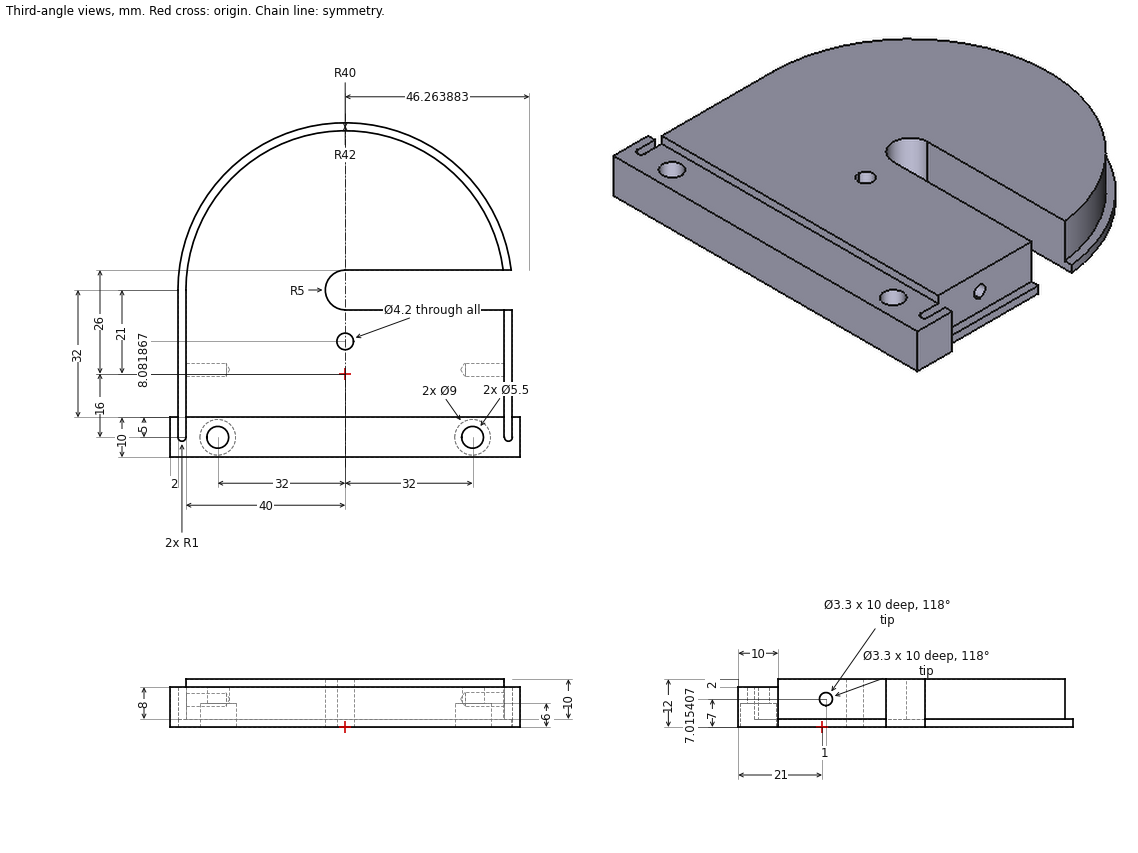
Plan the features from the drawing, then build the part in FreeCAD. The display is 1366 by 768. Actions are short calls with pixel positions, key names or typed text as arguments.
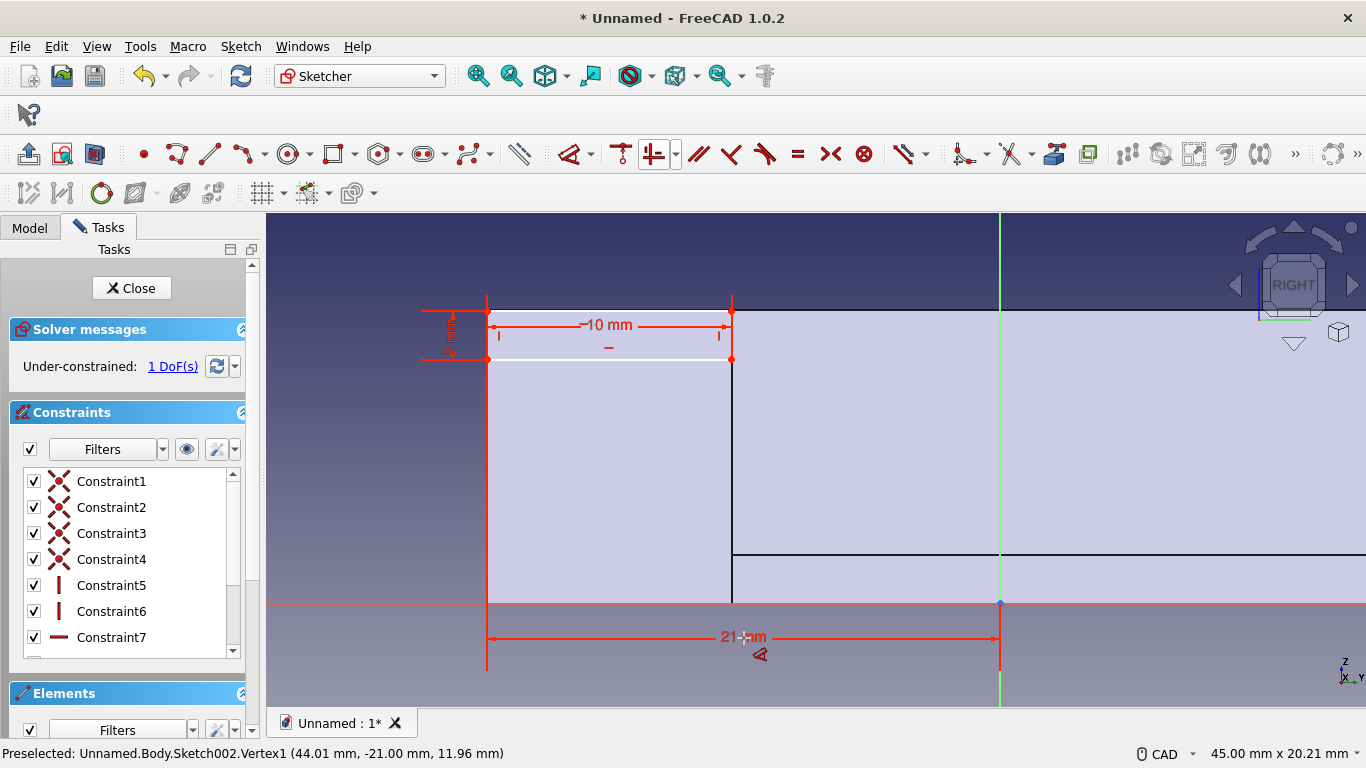
click(487, 311)
click(1034, 457)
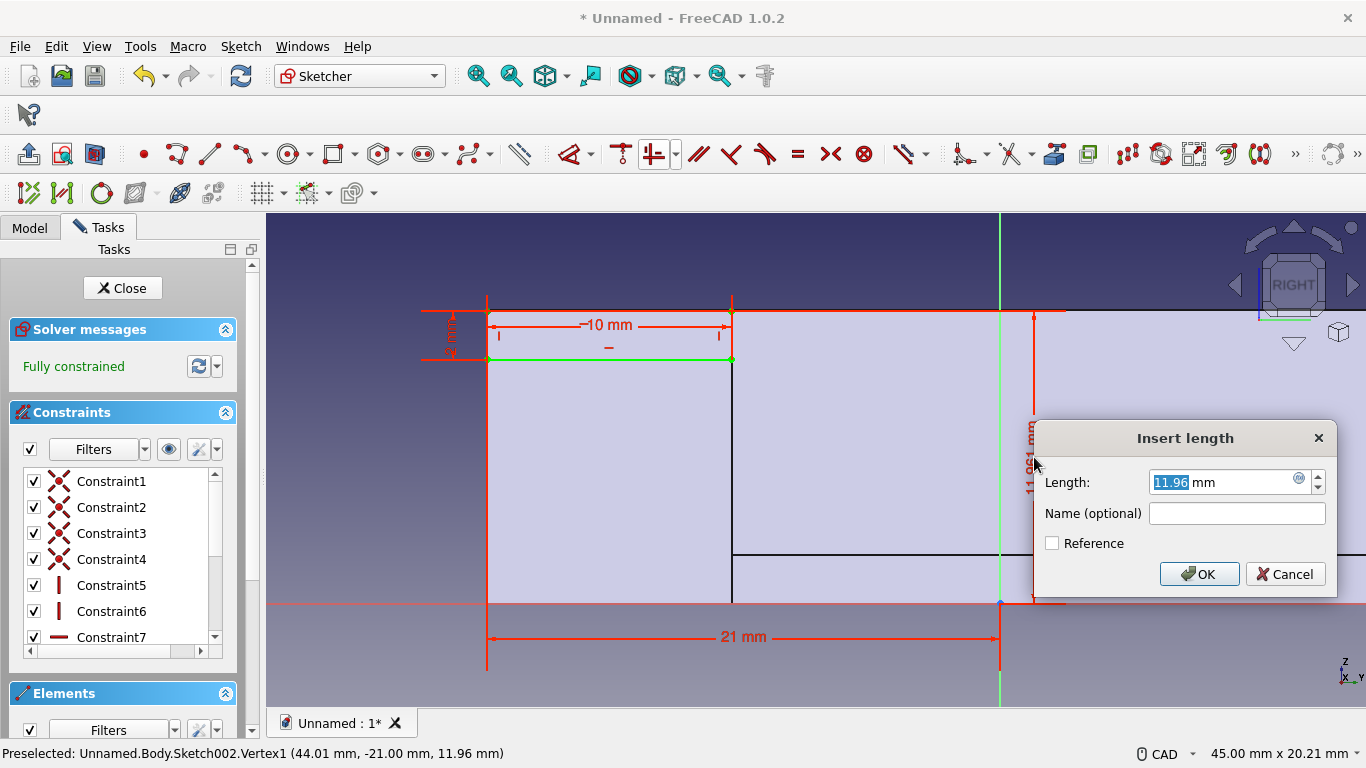
text(12)
key(Return)
key(Escape)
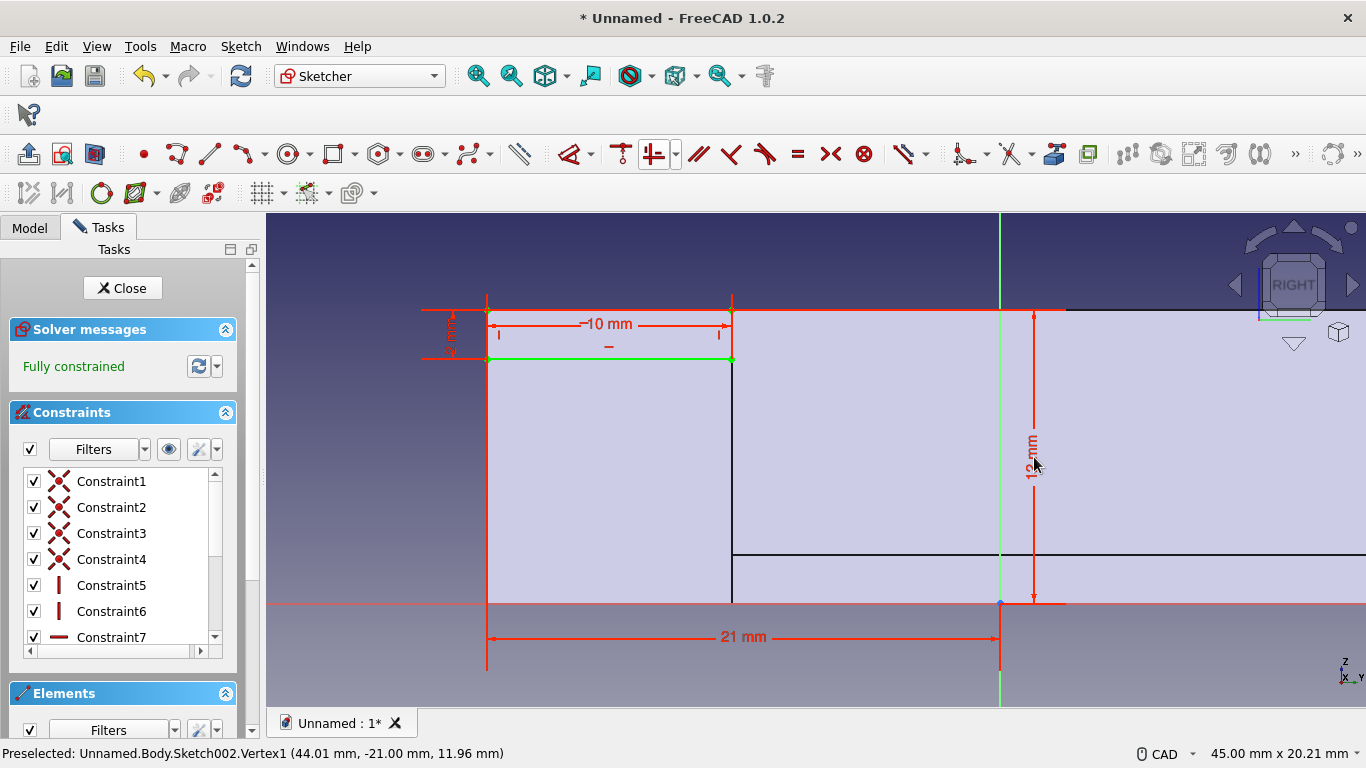
click(123, 288)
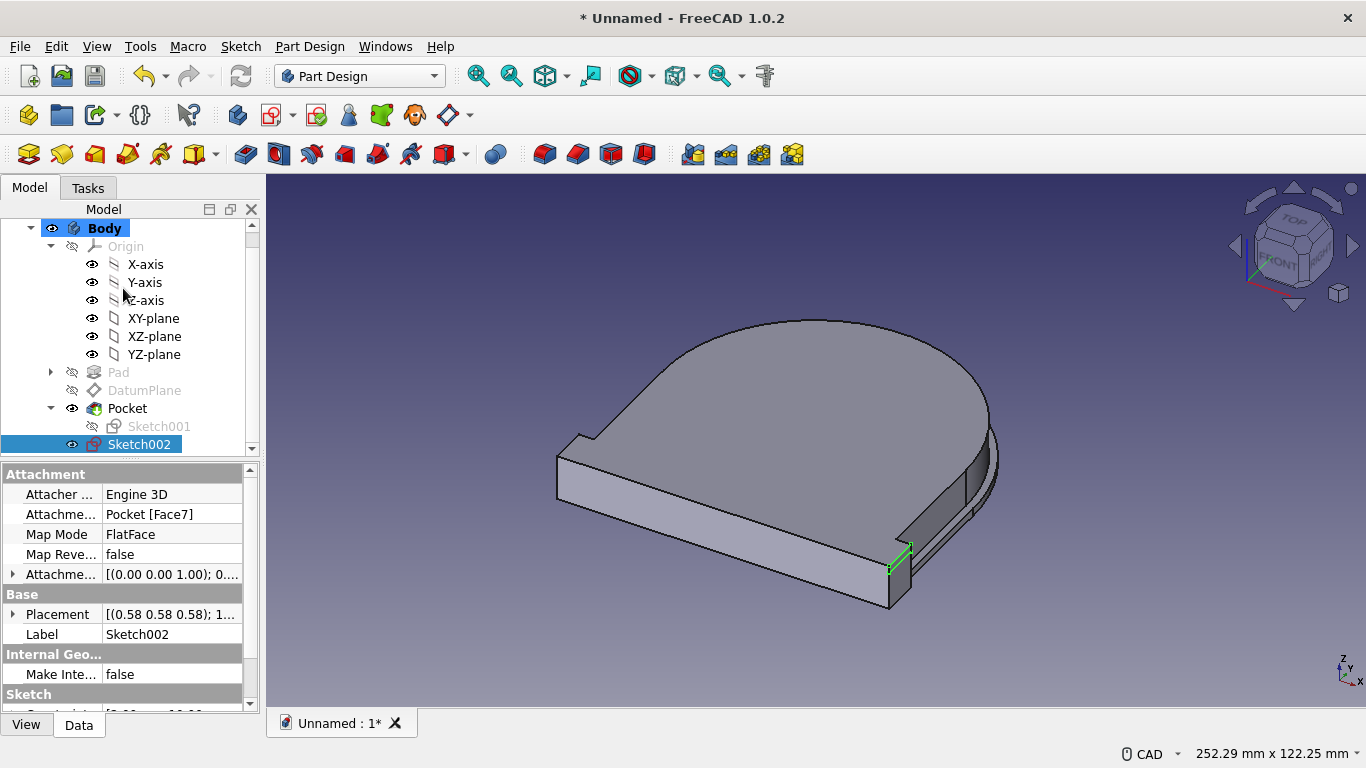
click(246, 154)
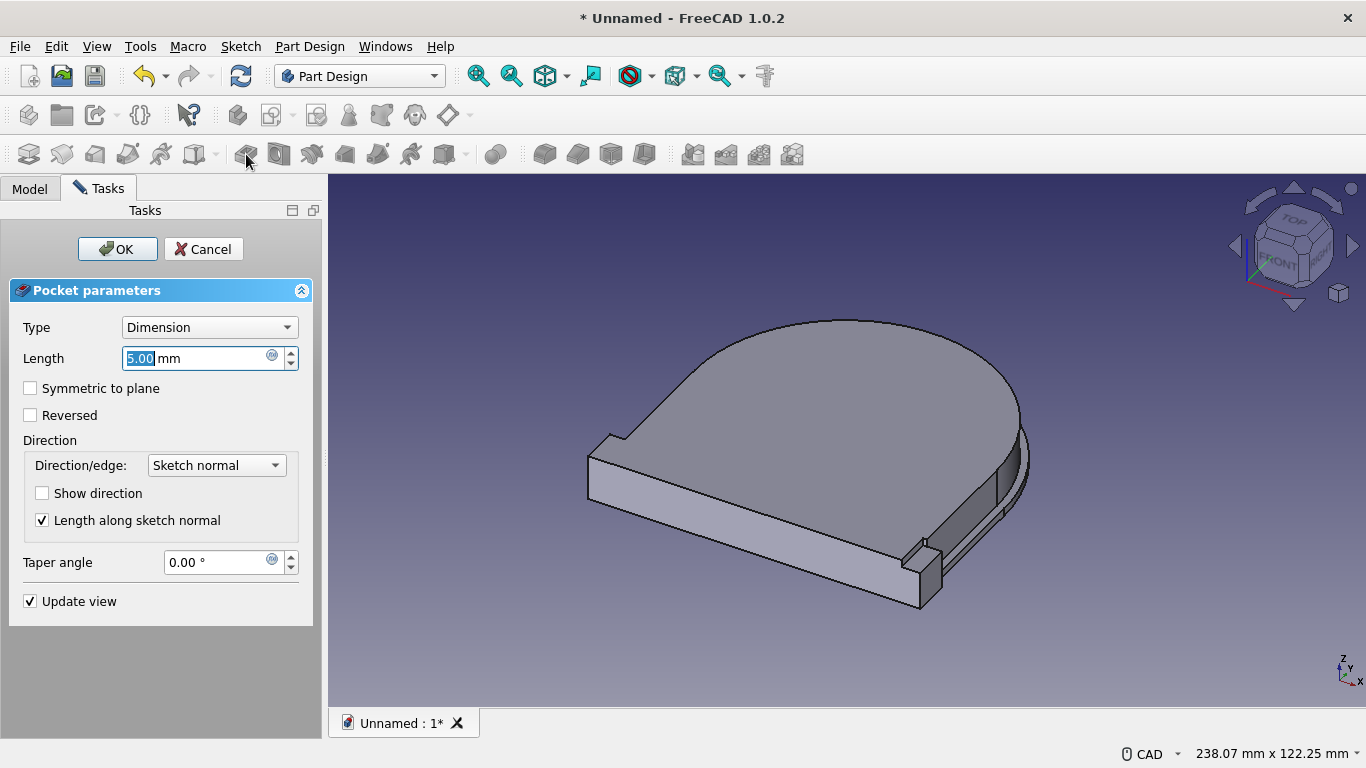
click(210, 328)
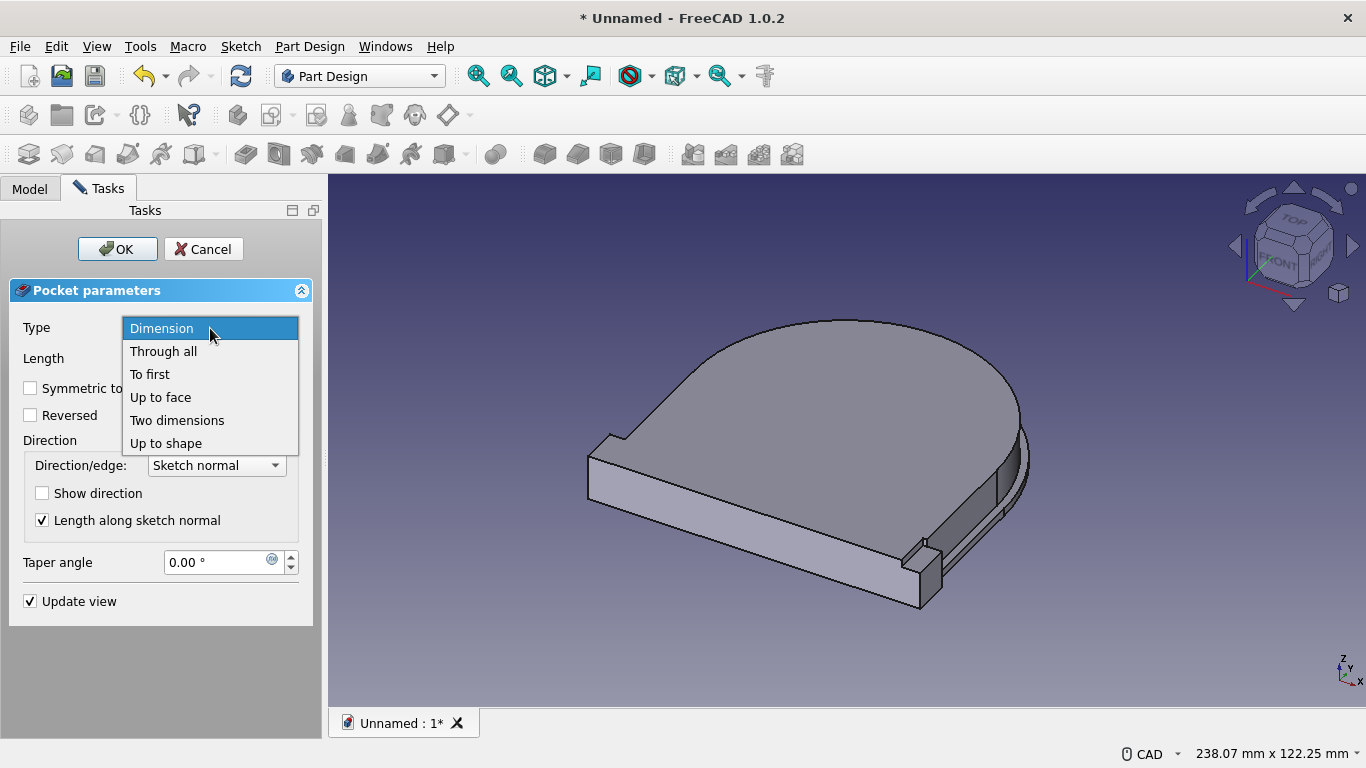
click(208, 352)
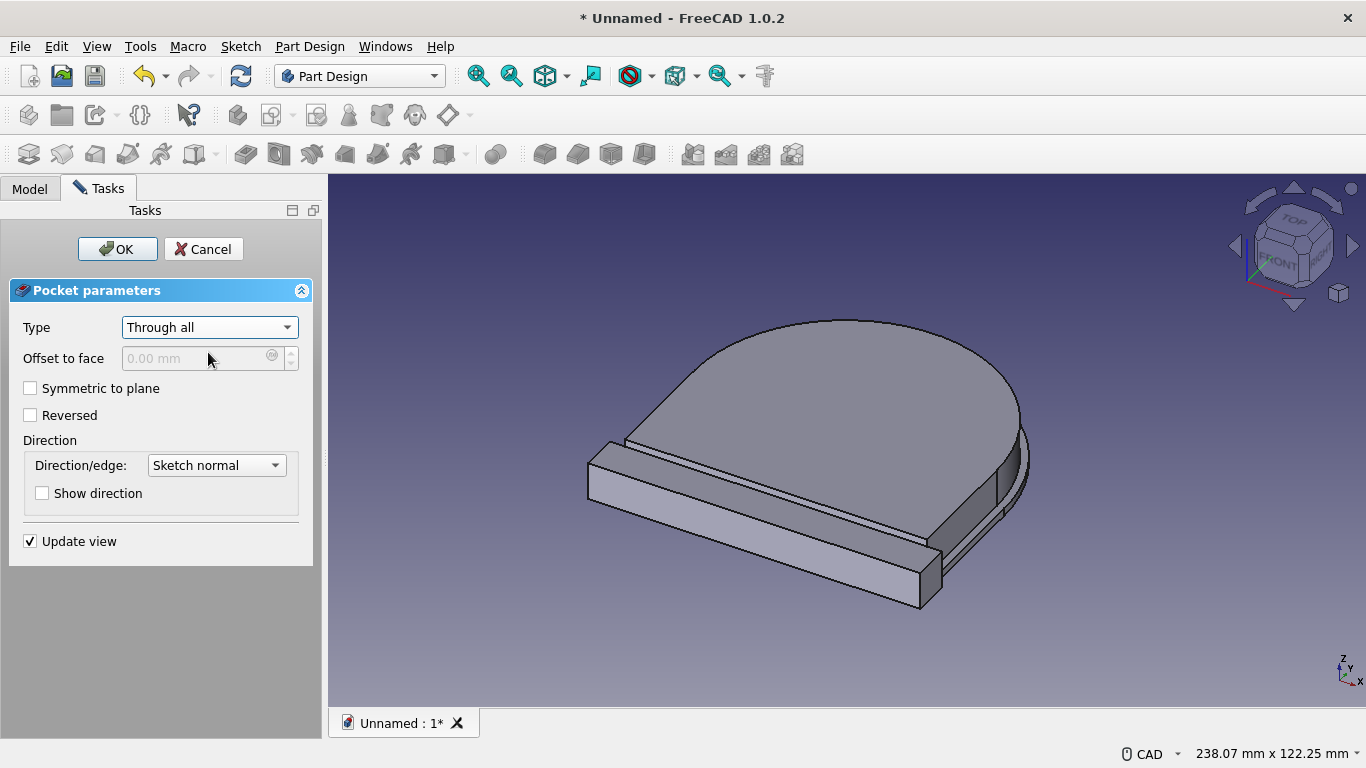
click(118, 249)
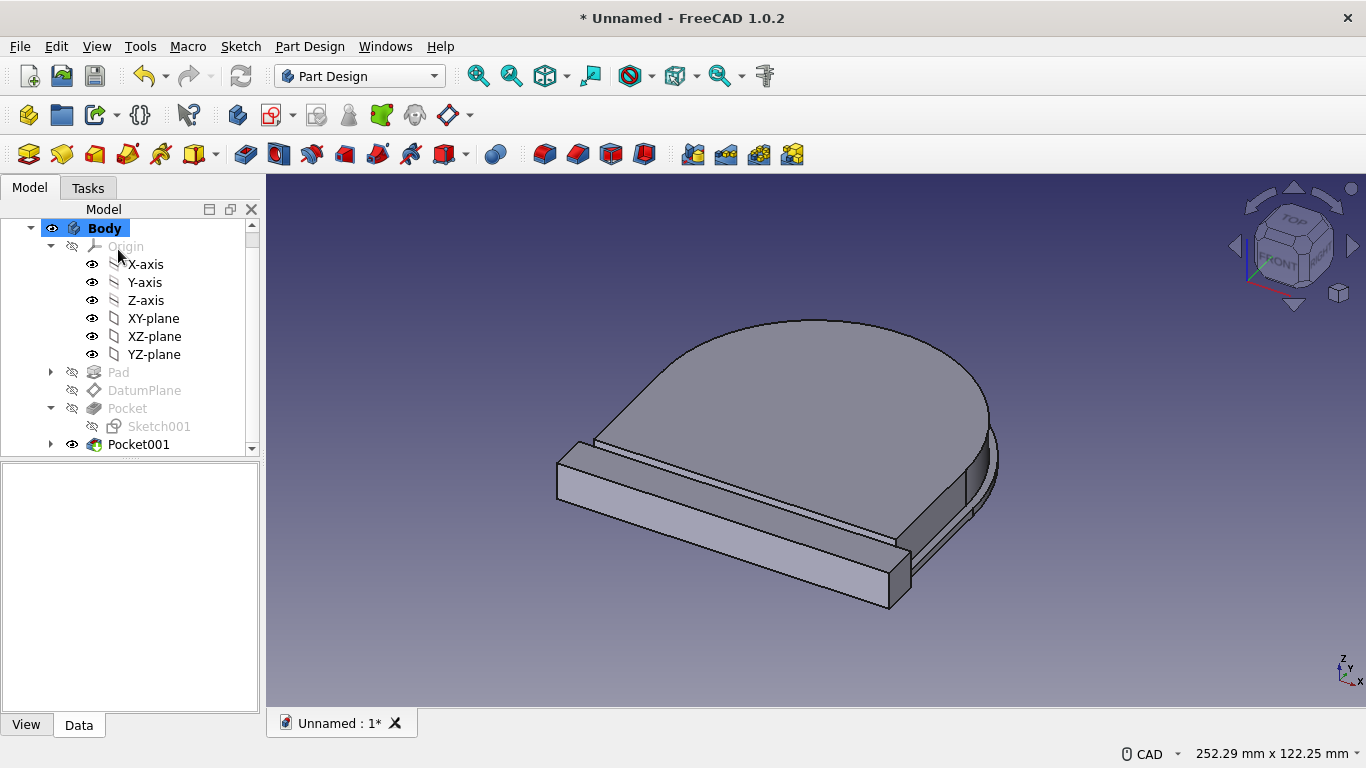
click(877, 554)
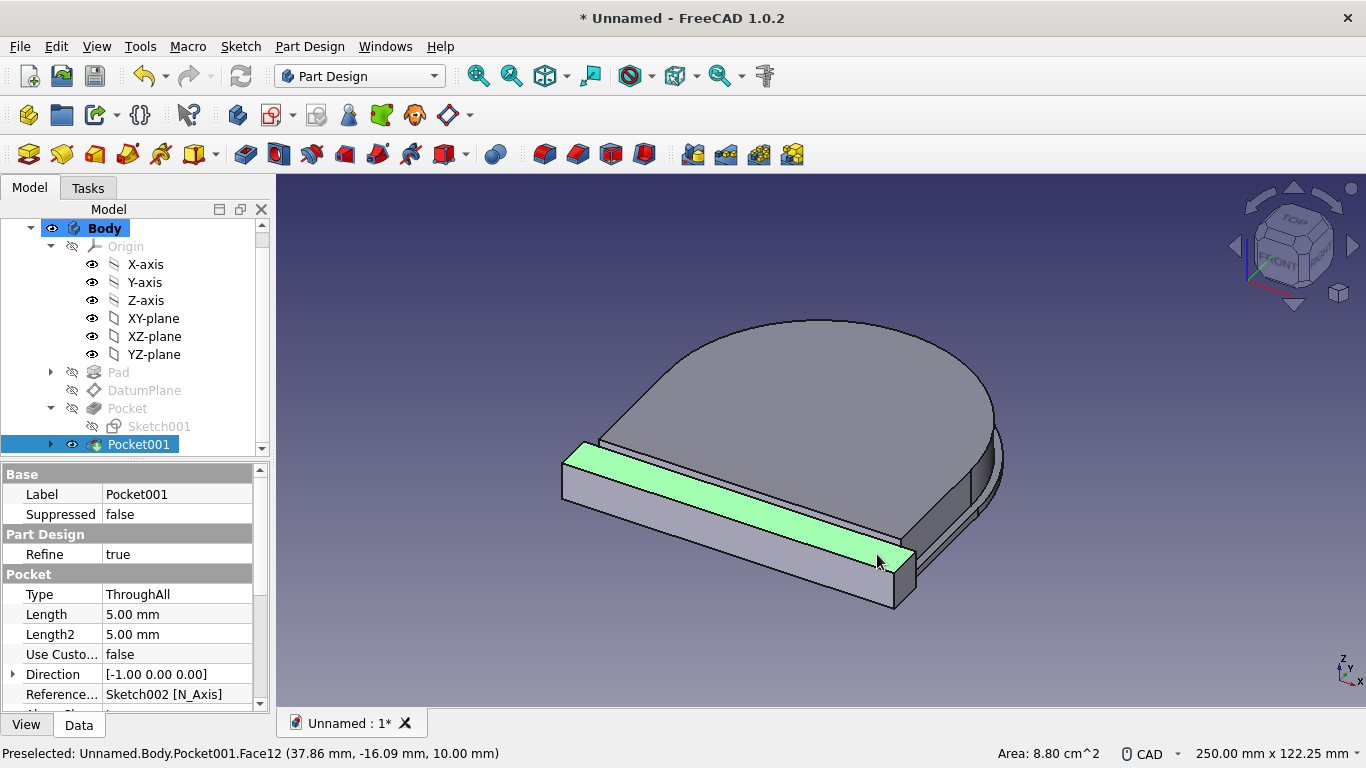
click(270, 116)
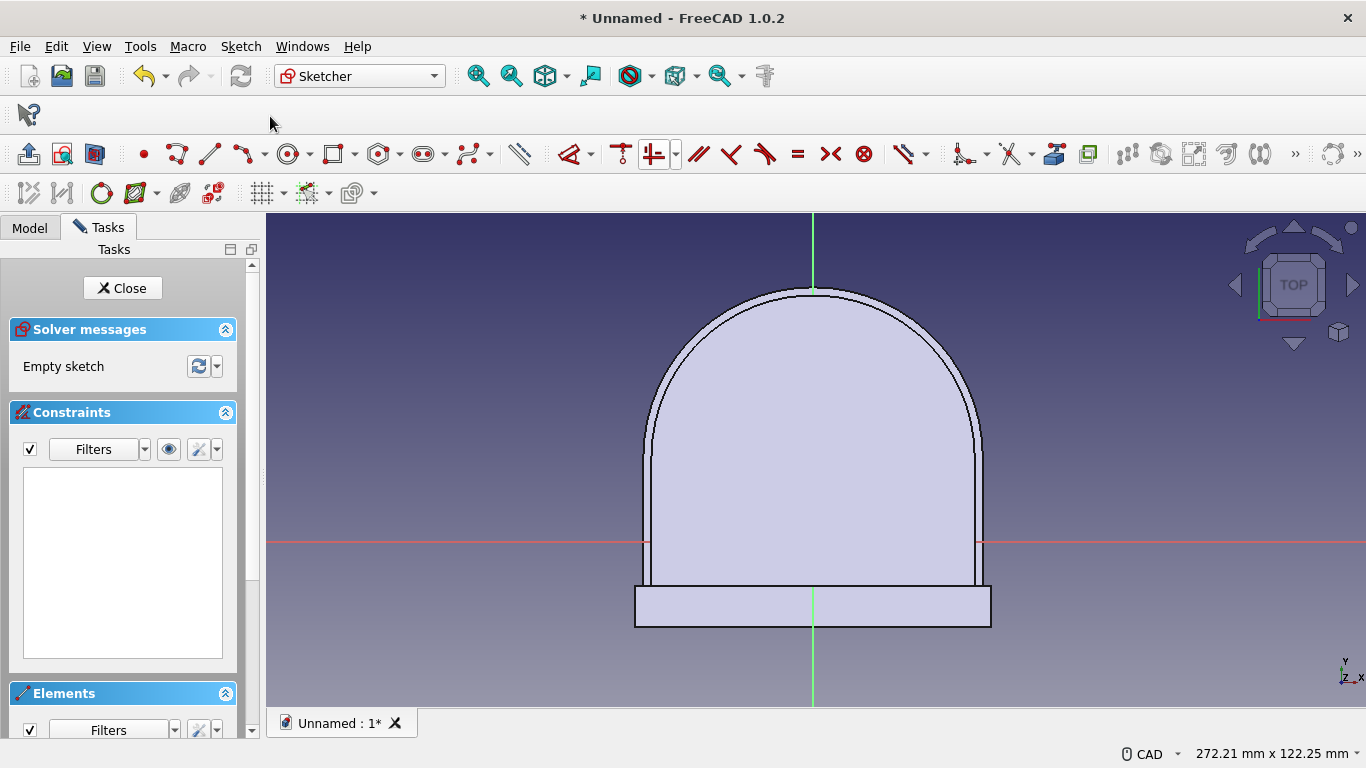
scroll(893, 679, up, 3)